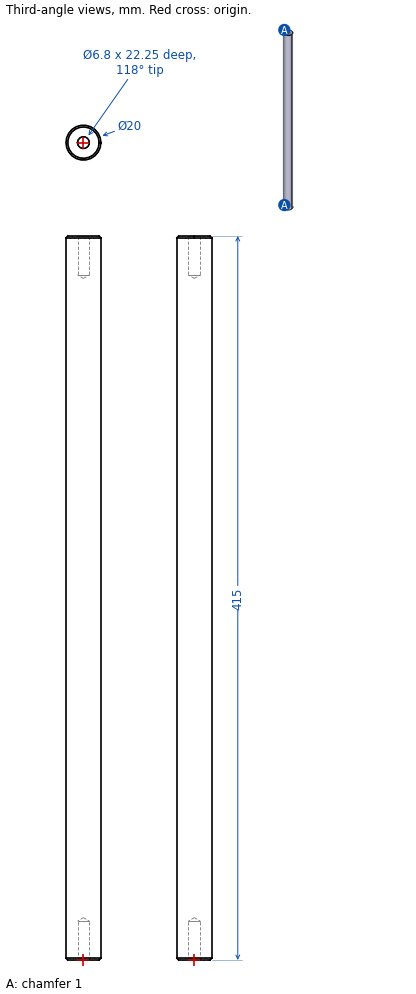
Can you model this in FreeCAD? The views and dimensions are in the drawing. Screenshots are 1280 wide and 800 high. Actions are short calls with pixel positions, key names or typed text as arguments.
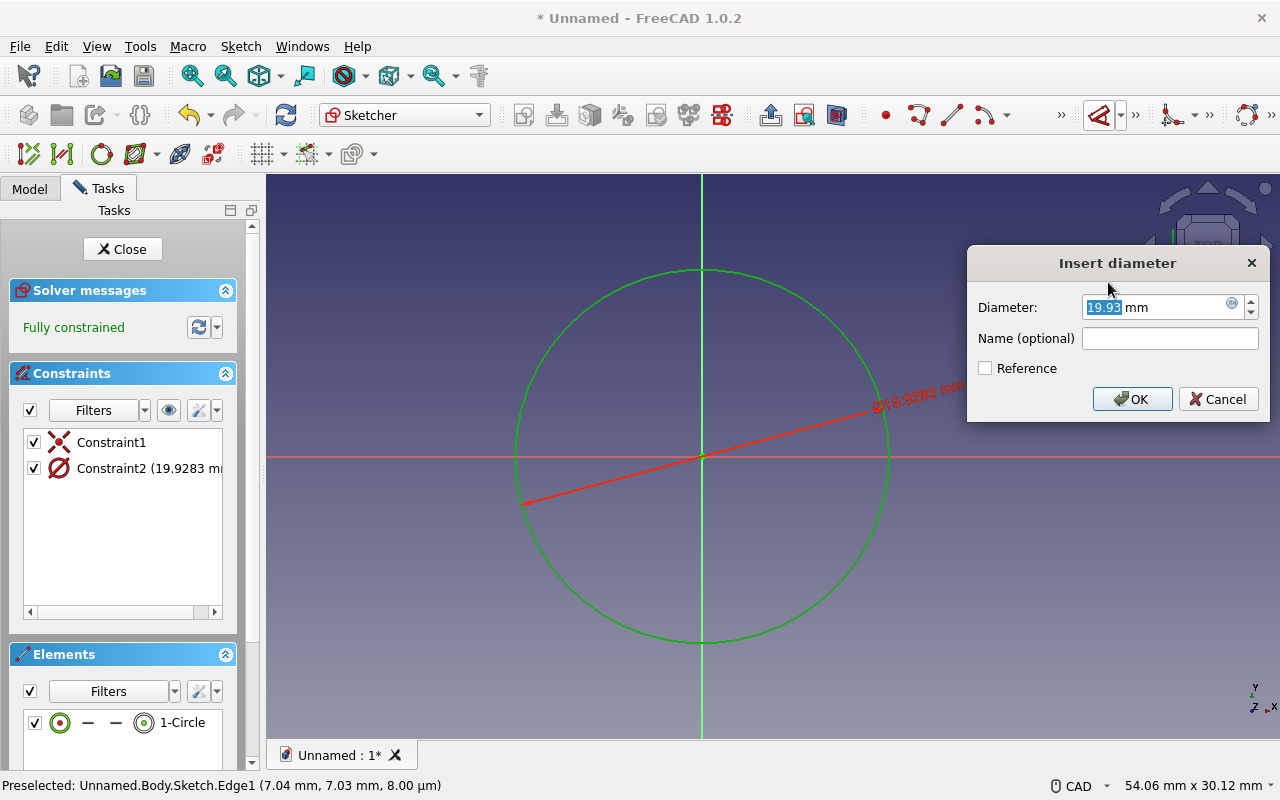
text(20)
key(Return)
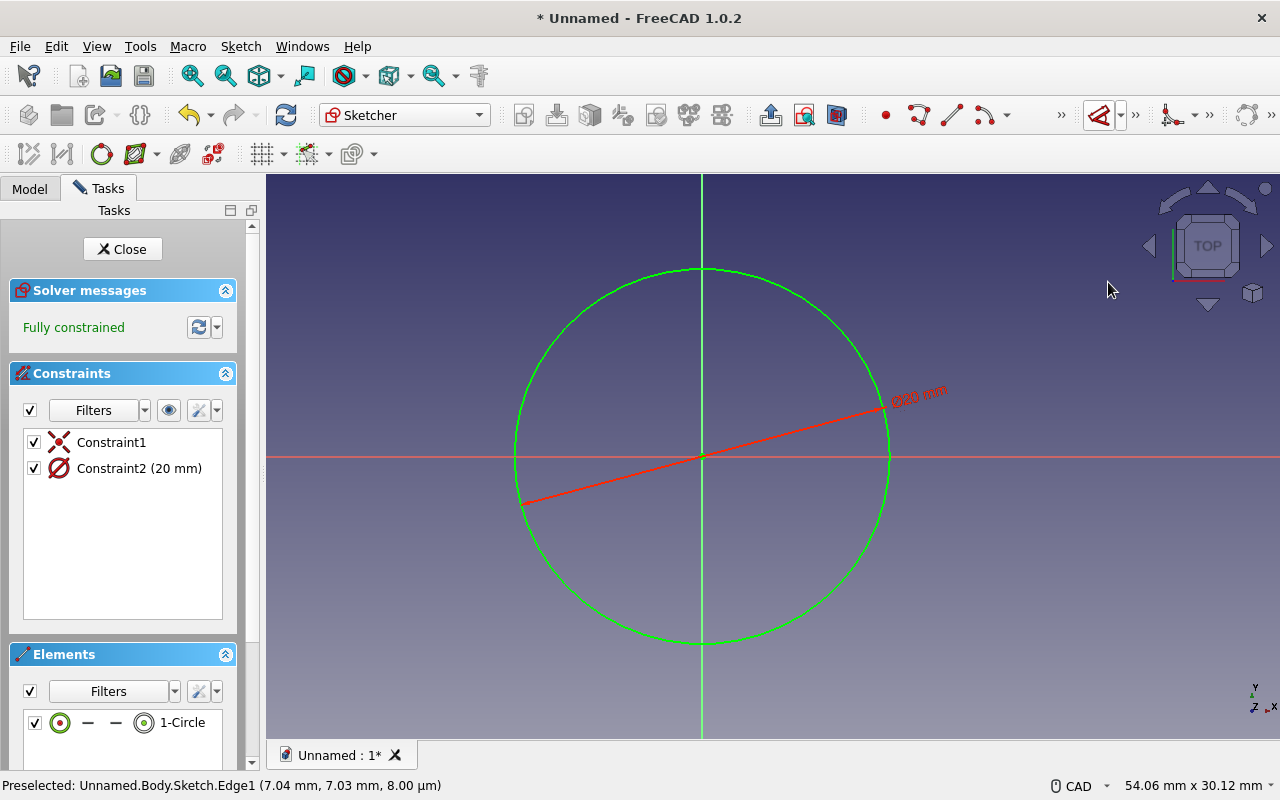
click(123, 249)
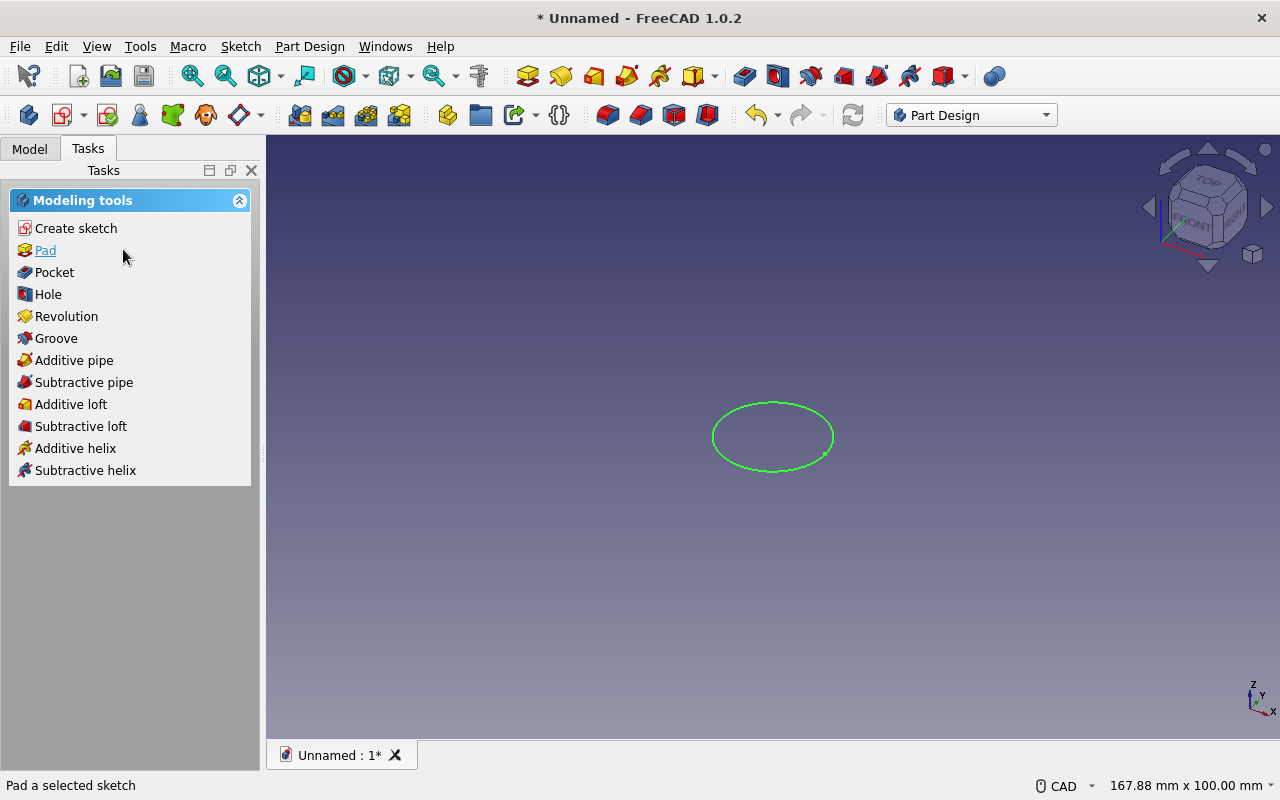
click(528, 76)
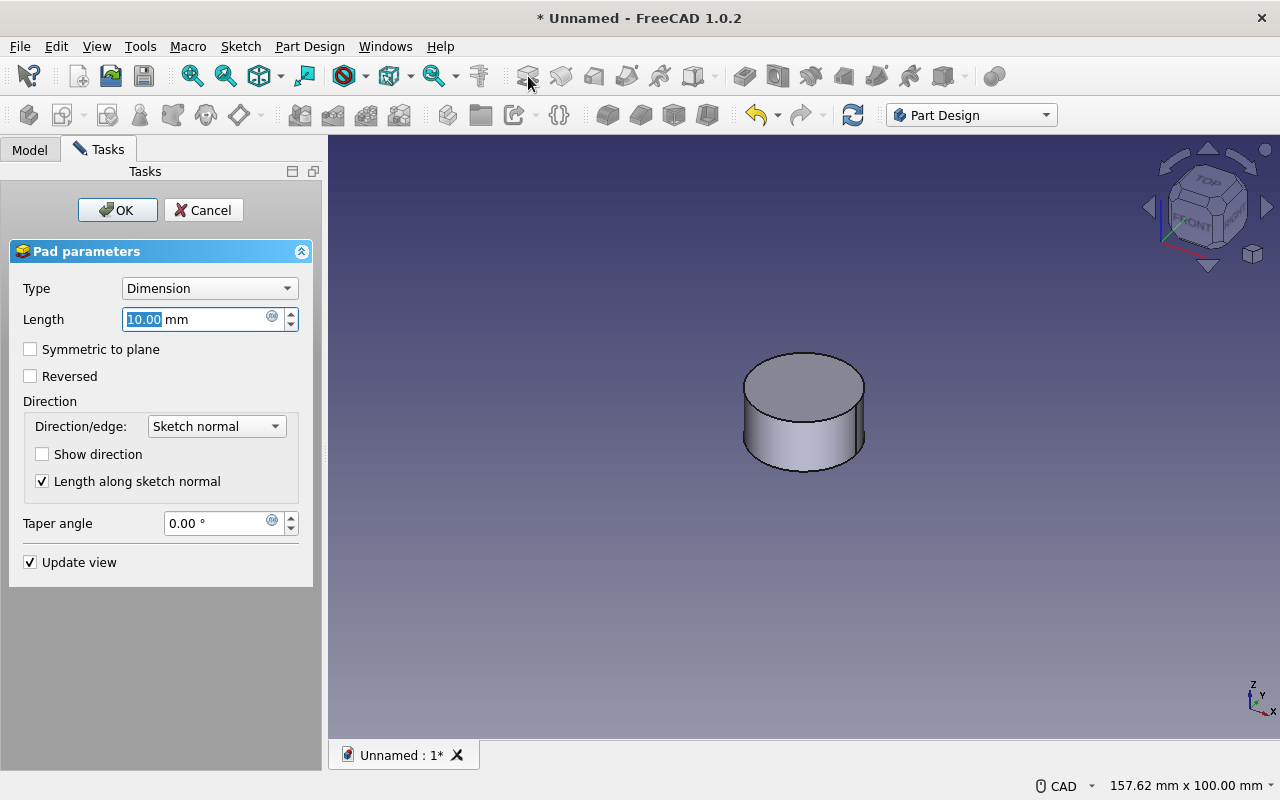
text(415)
key(Tab)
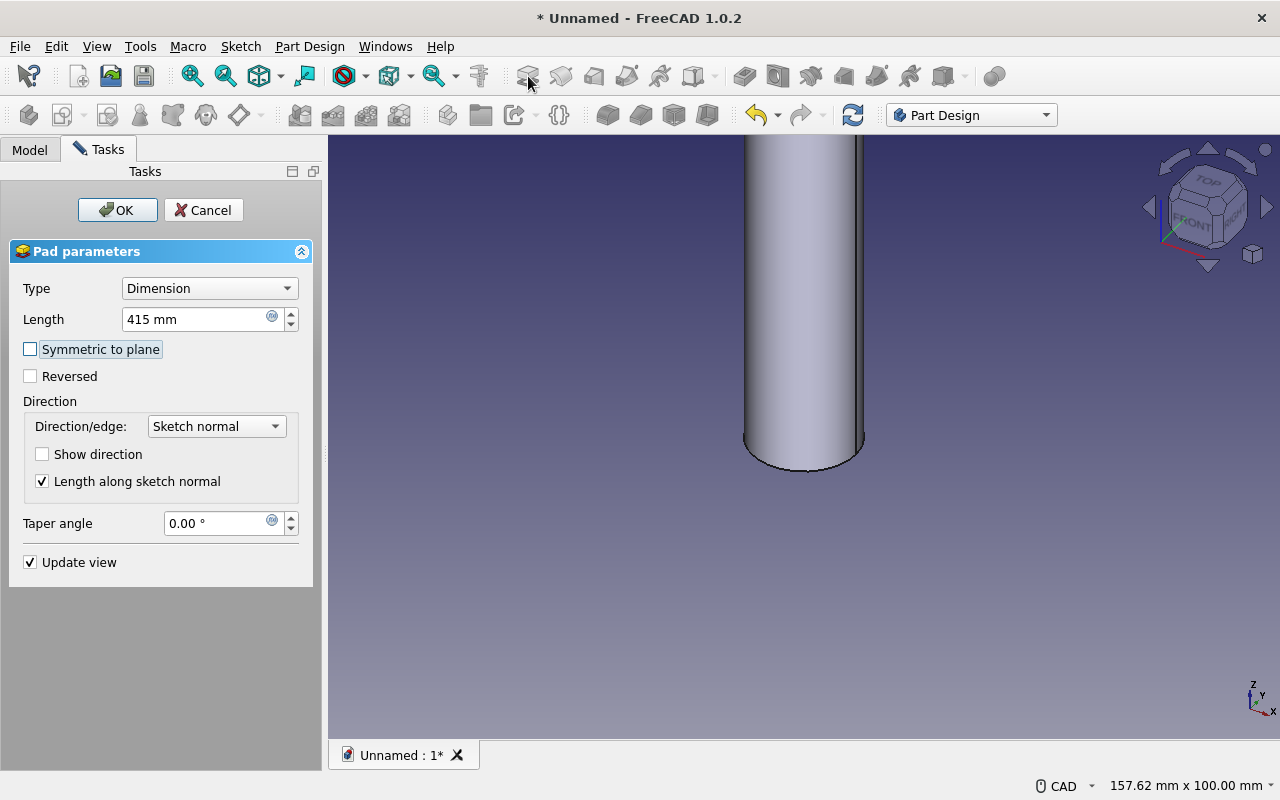
click(118, 210)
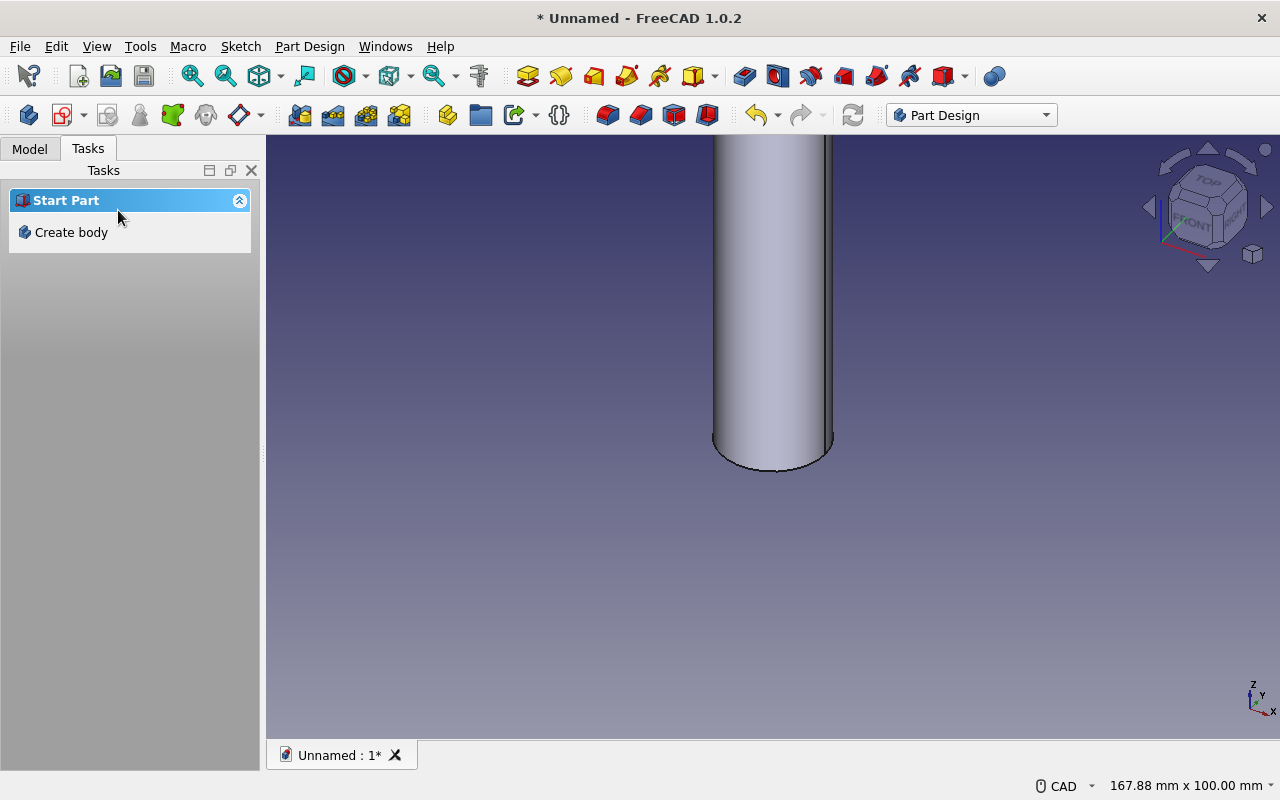
click(193, 76)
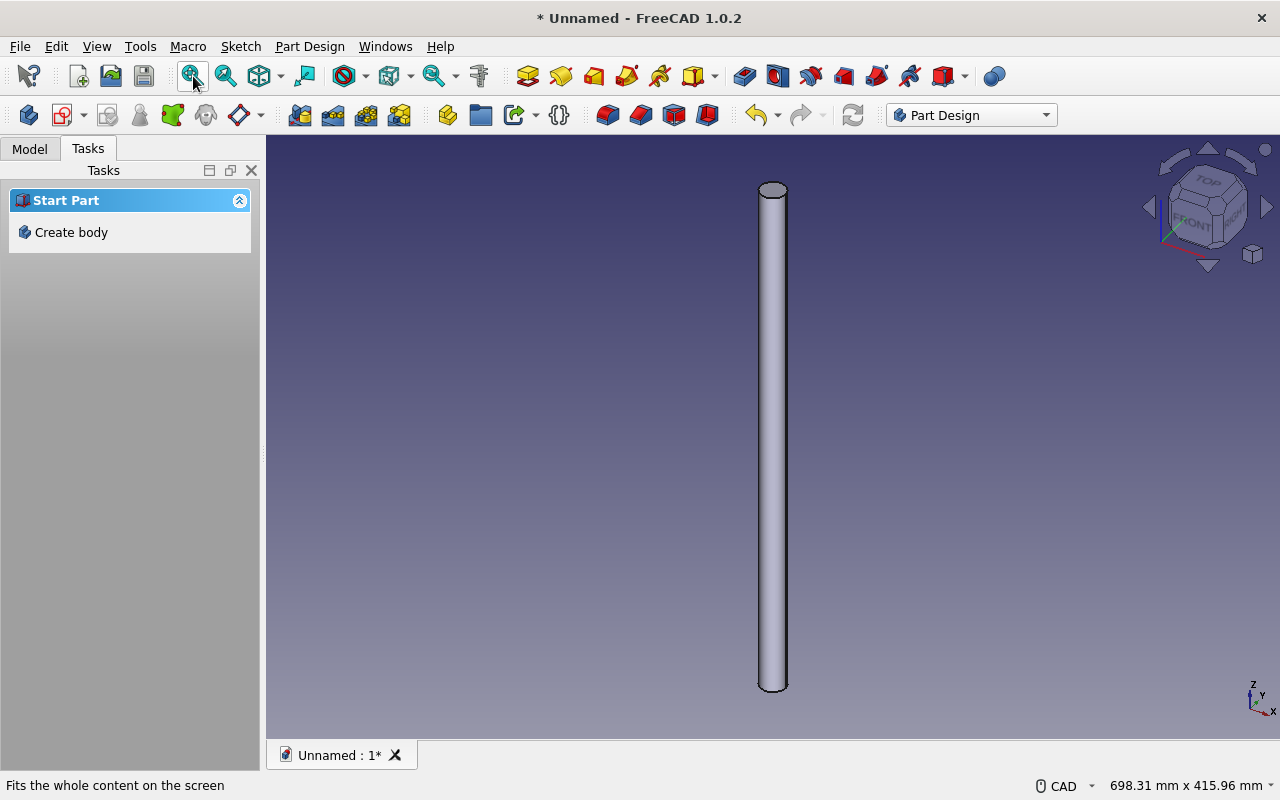
click(773, 189)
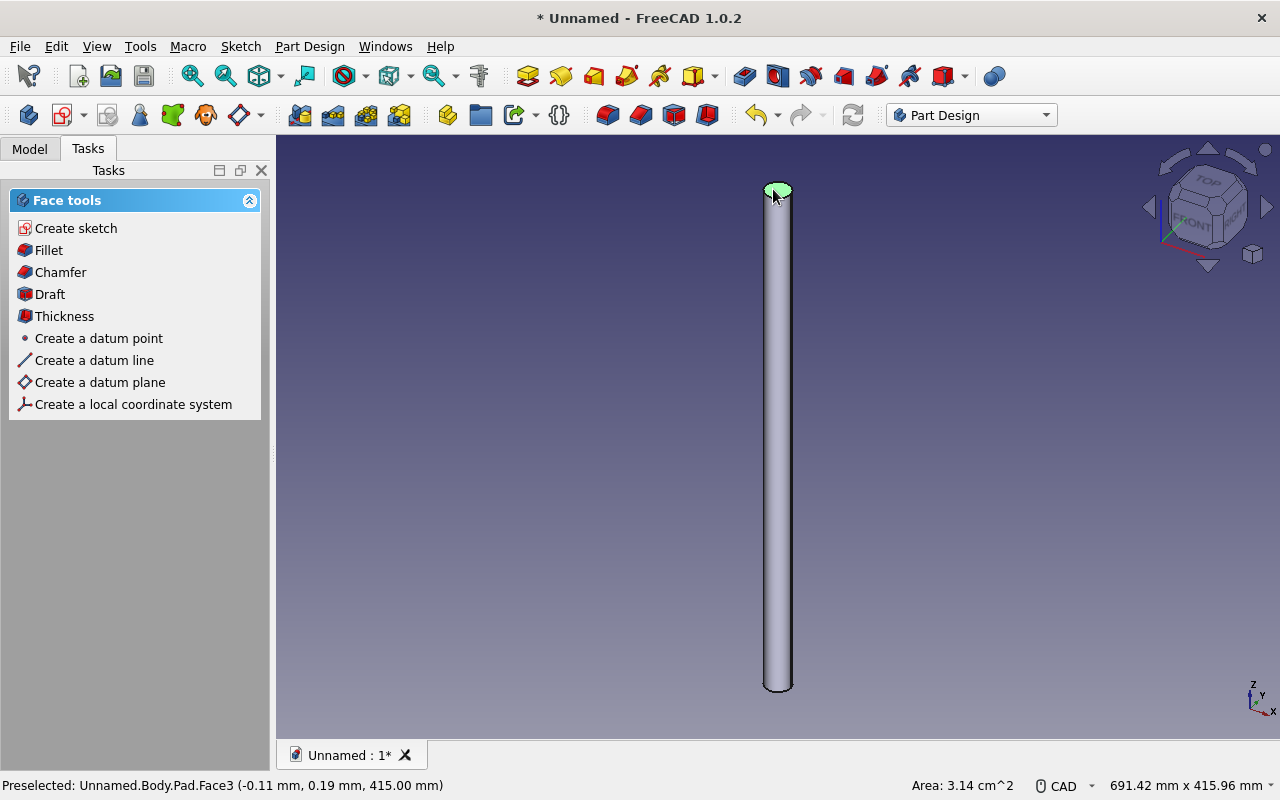
click(62, 116)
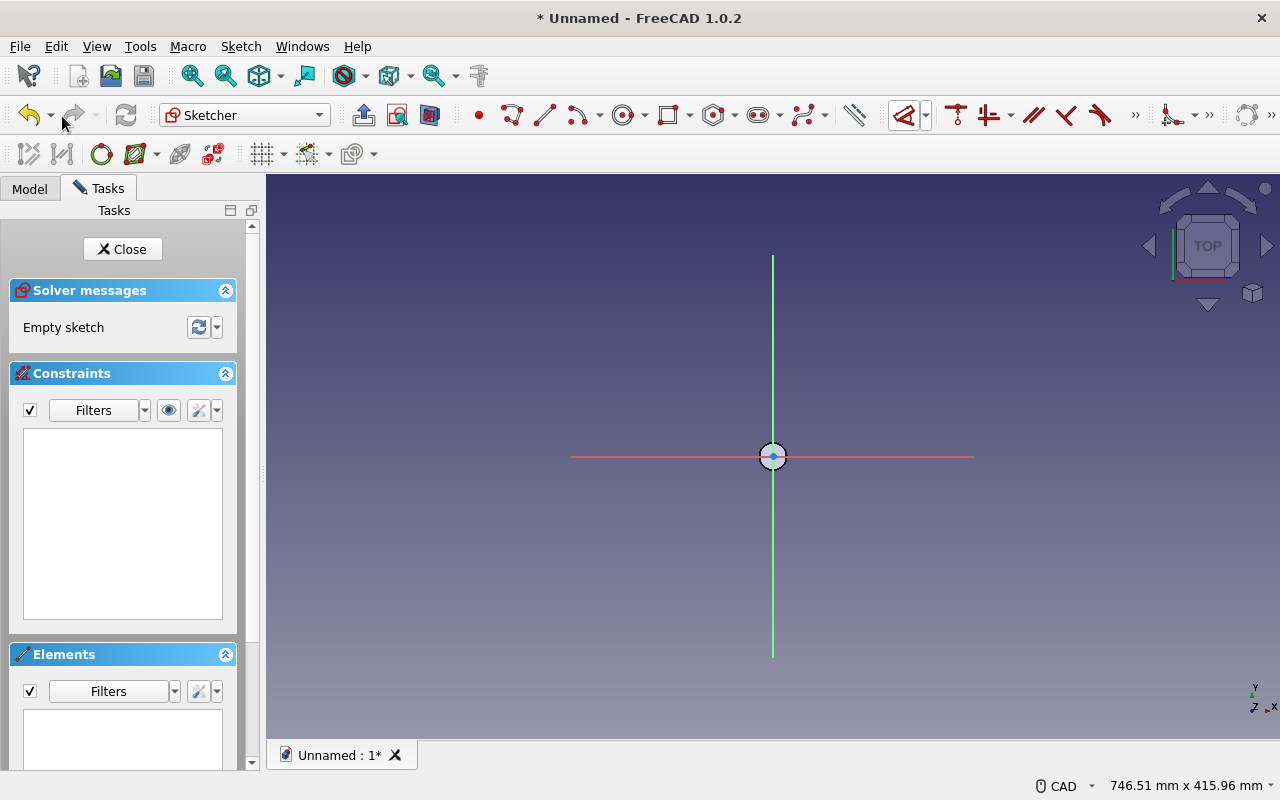
scroll(777, 457, up, 15)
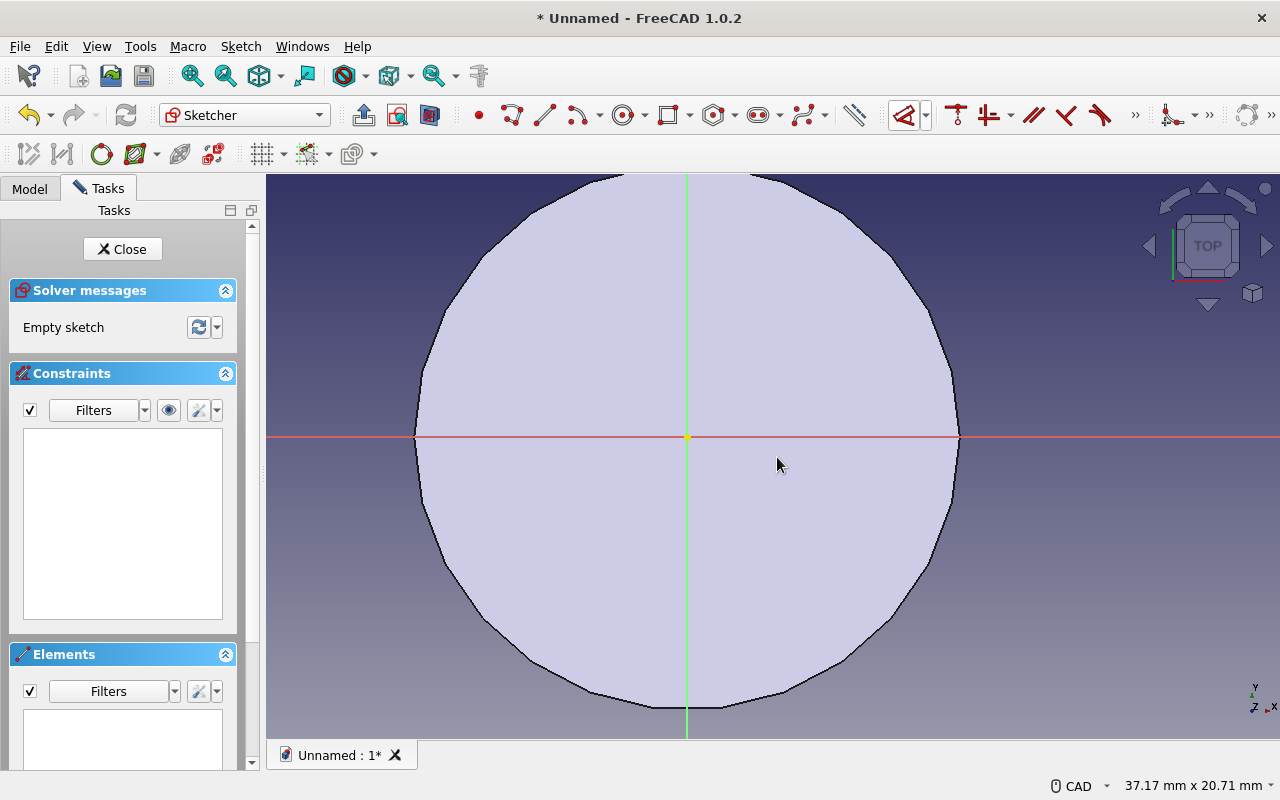
scroll(666, 414, up, 3)